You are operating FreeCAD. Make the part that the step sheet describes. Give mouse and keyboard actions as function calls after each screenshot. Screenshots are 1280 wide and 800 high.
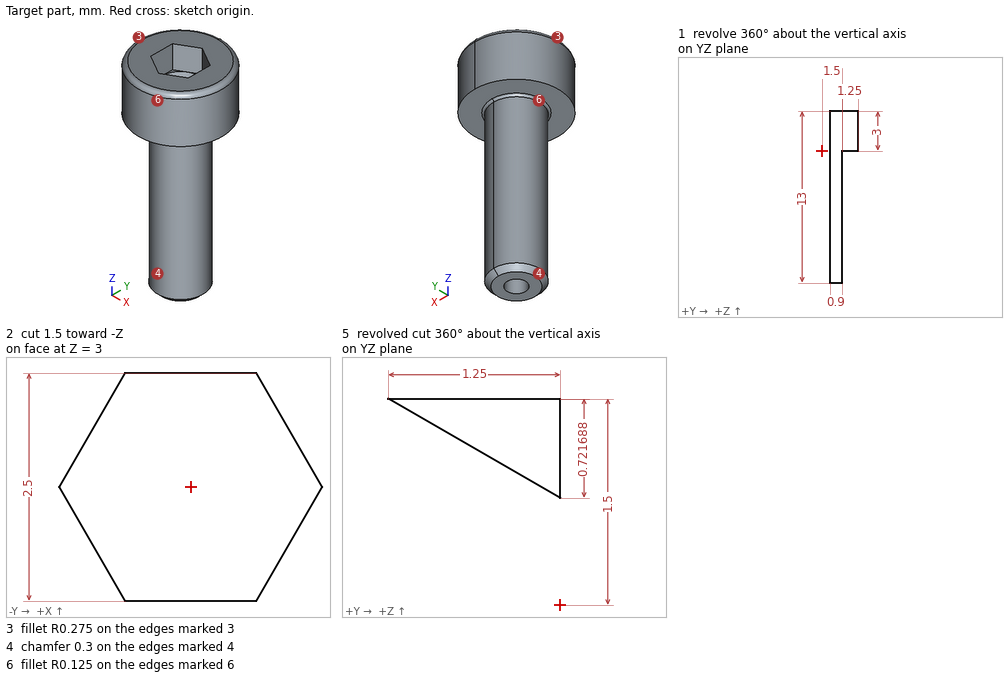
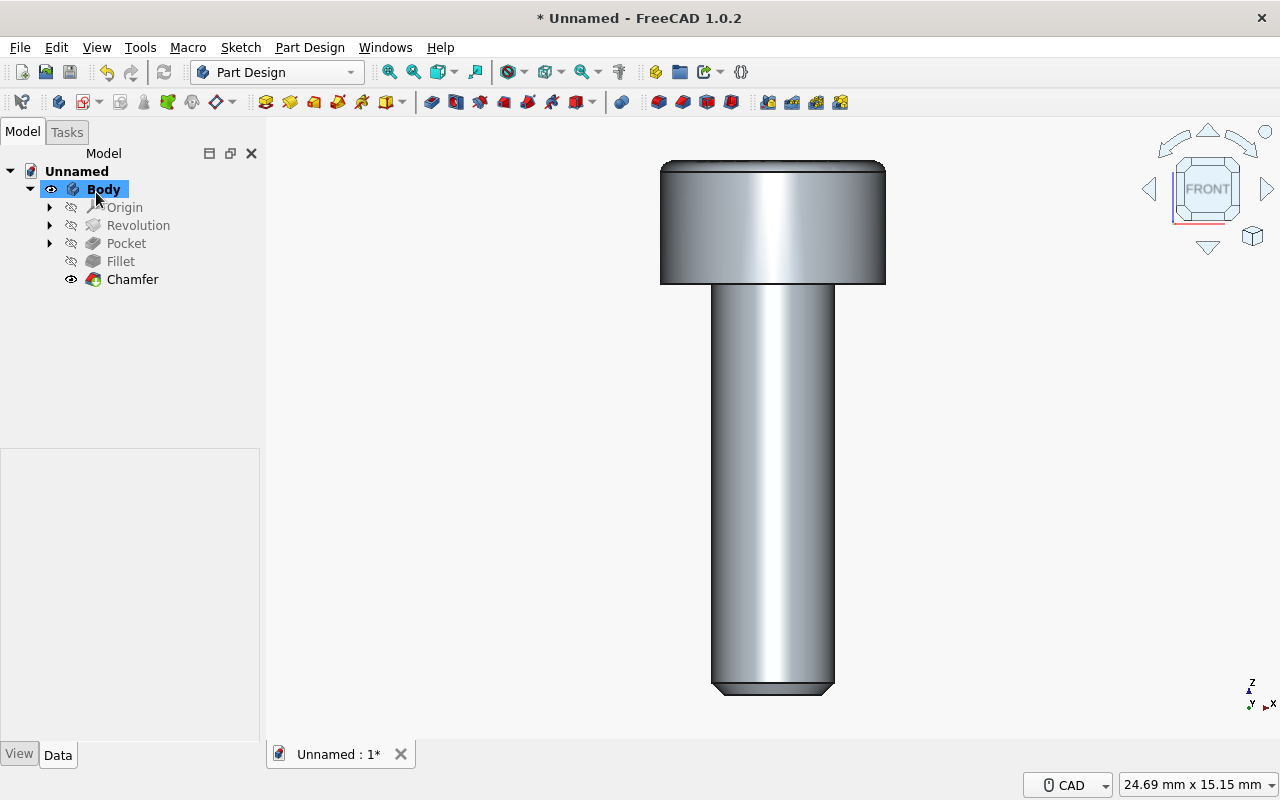
click(84, 102)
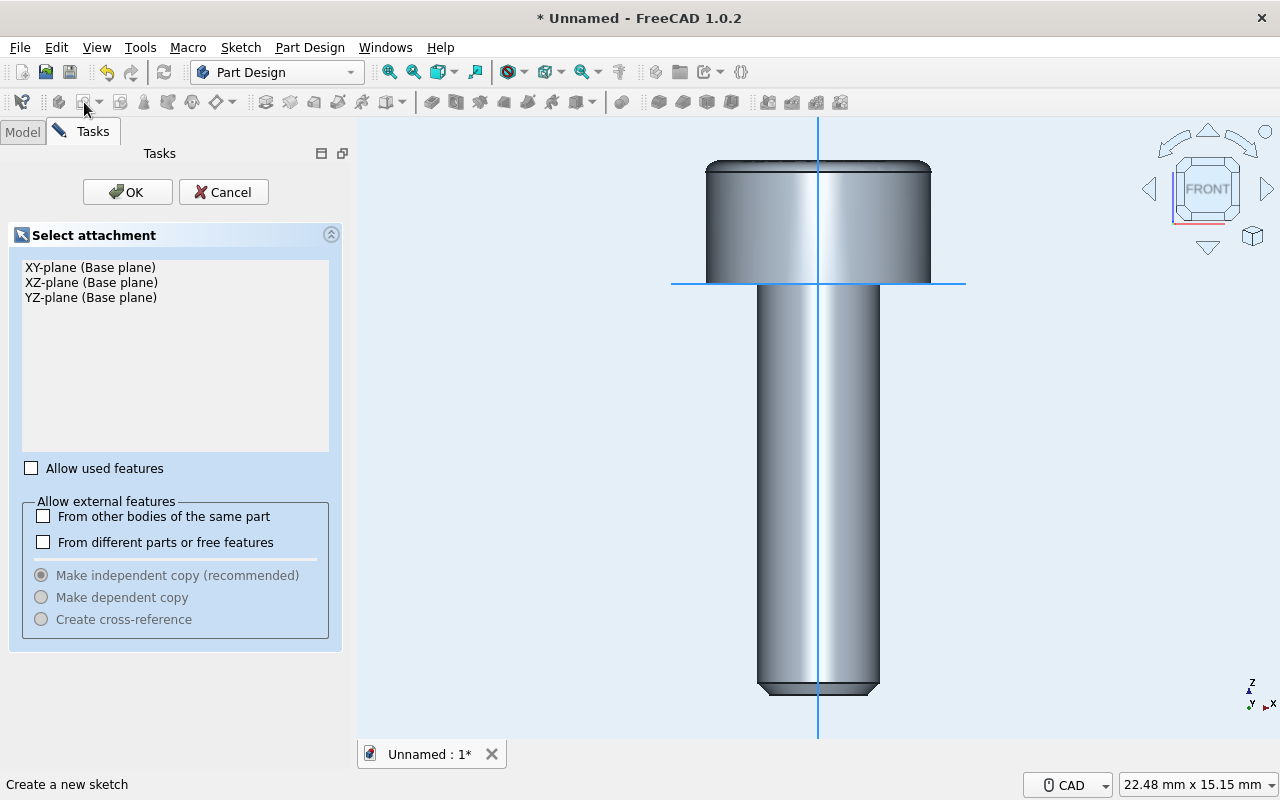
click(82, 298)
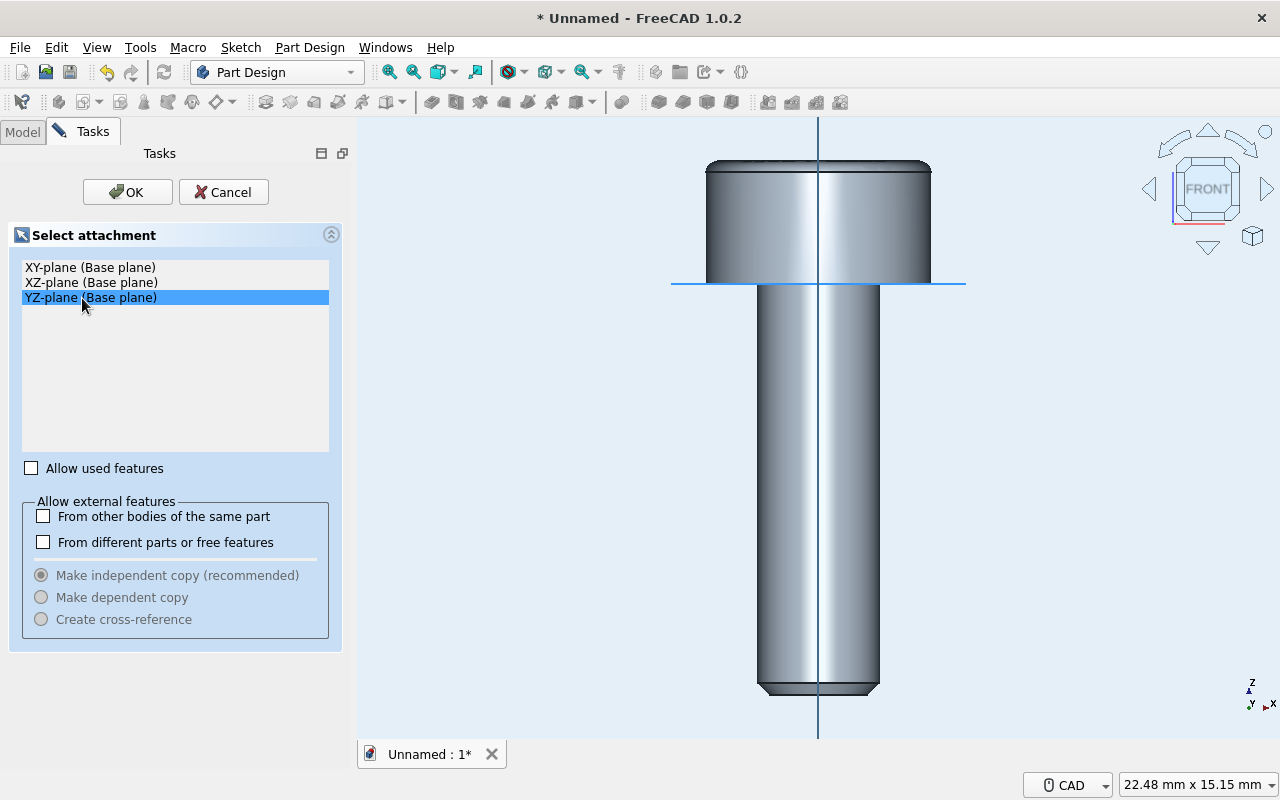
click(128, 192)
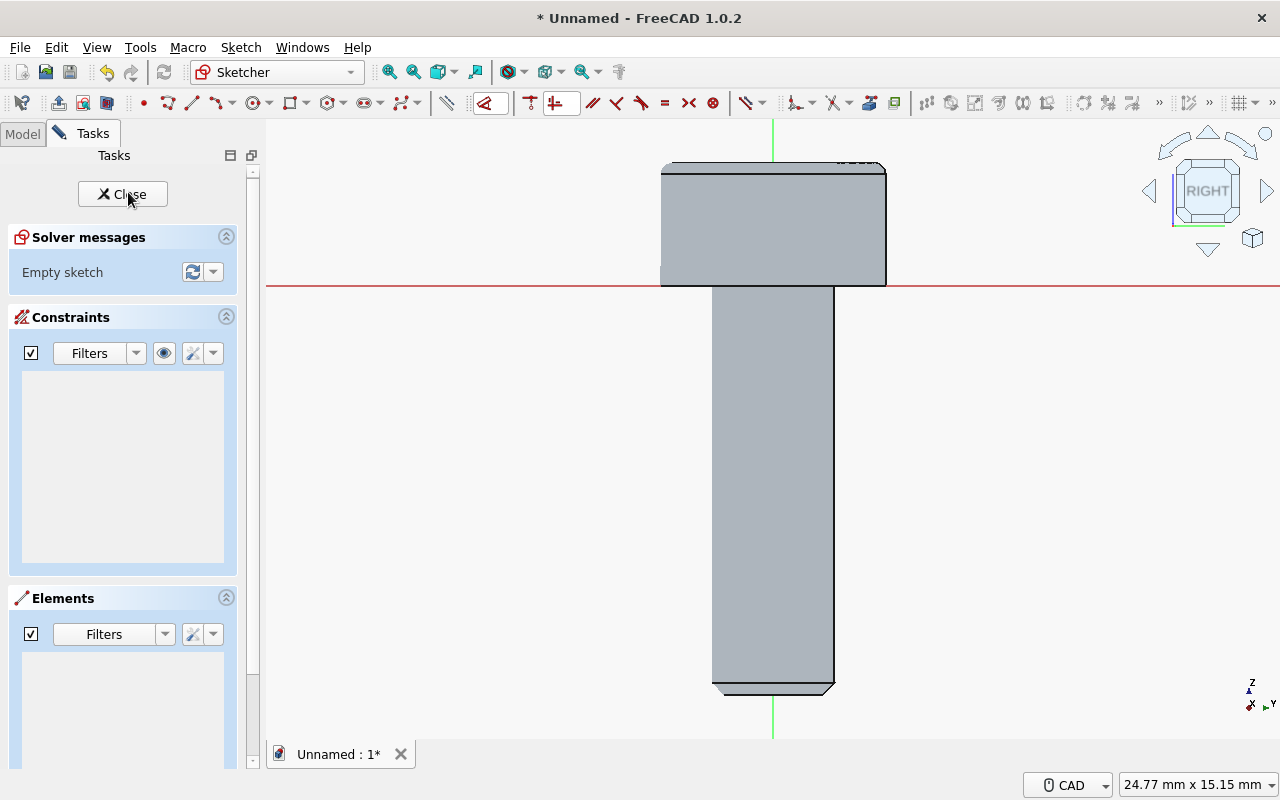
click(108, 104)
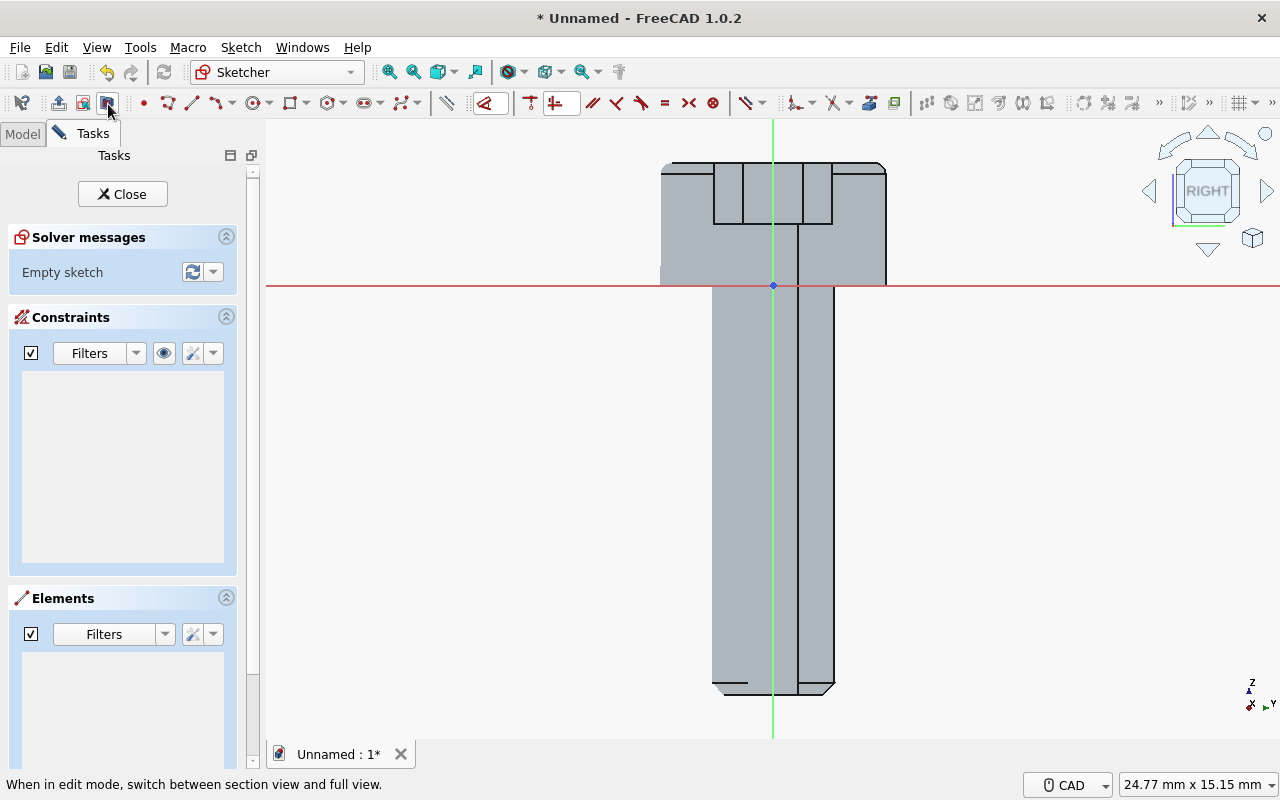
scroll(756, 221, up, 9)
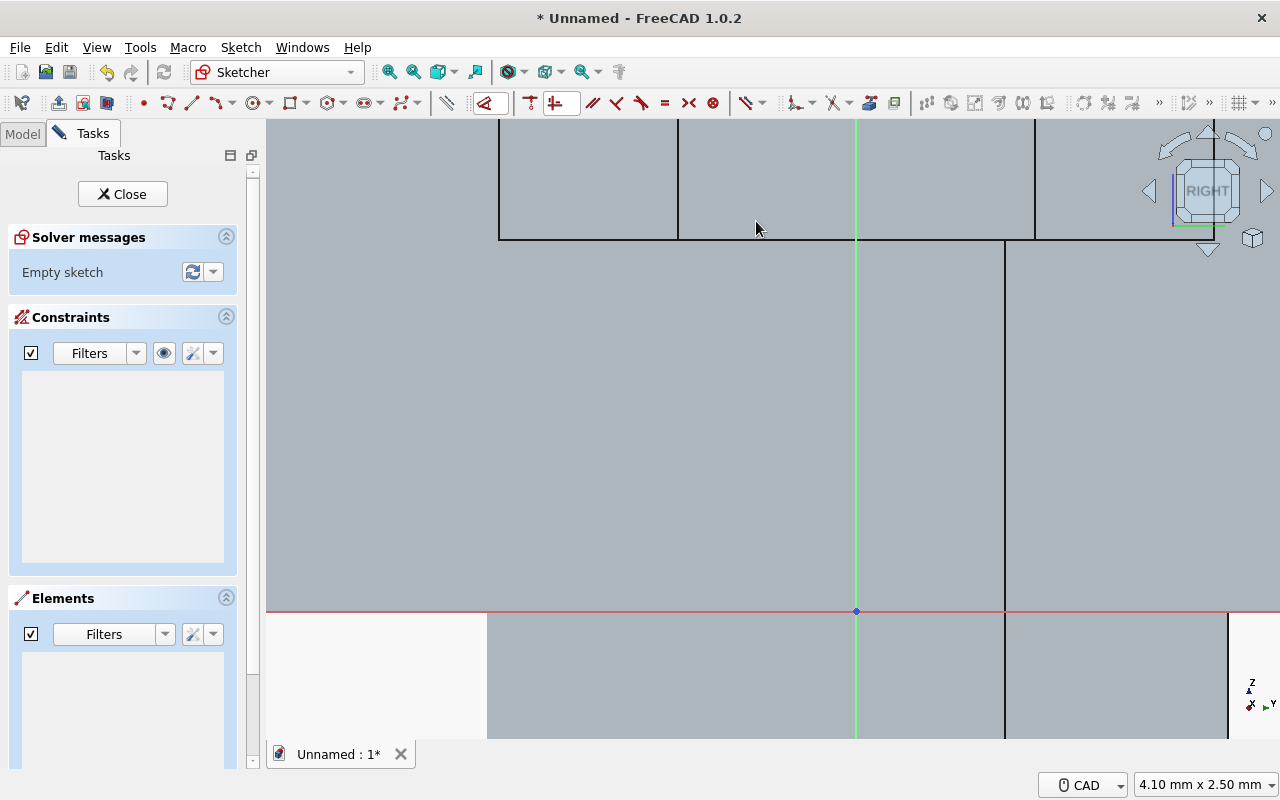
click(168, 104)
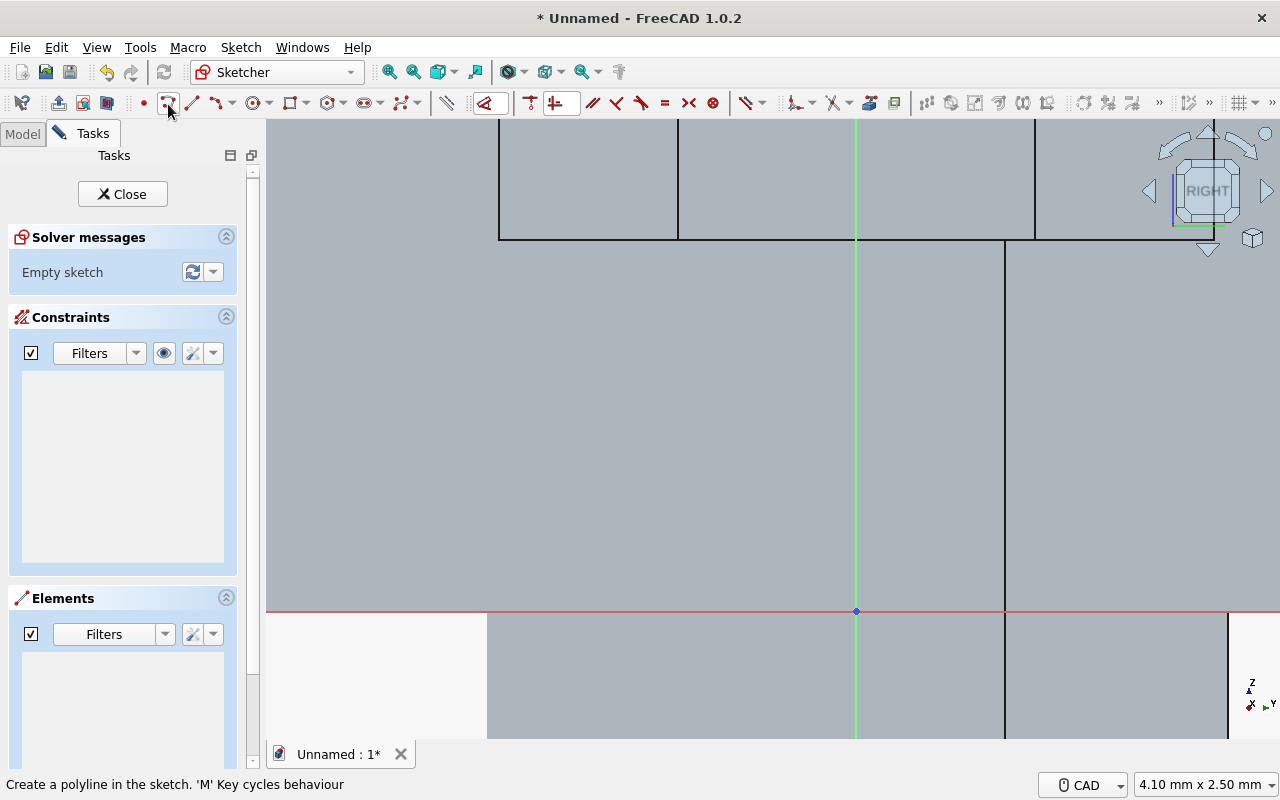
click(856, 419)
click(847, 240)
click(547, 240)
click(856, 420)
key(Escape)
key(Escape)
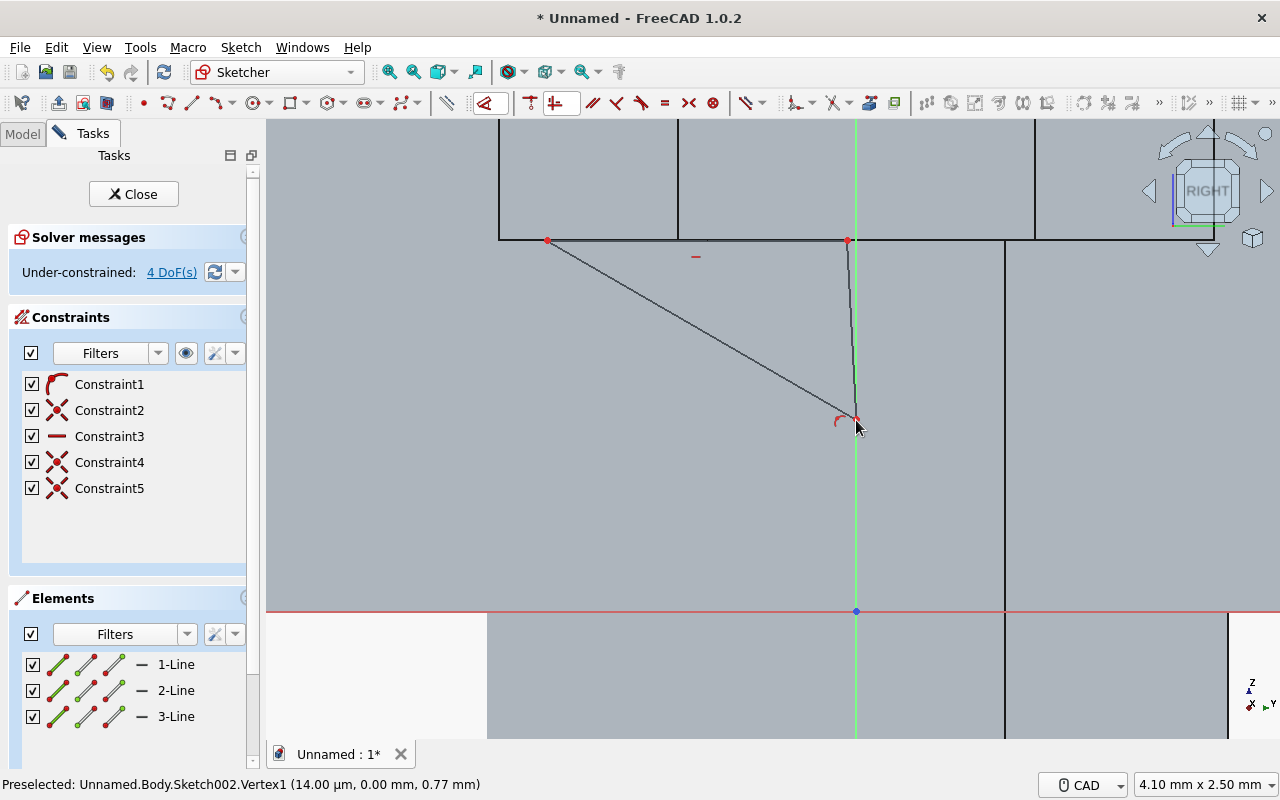
click(854, 366)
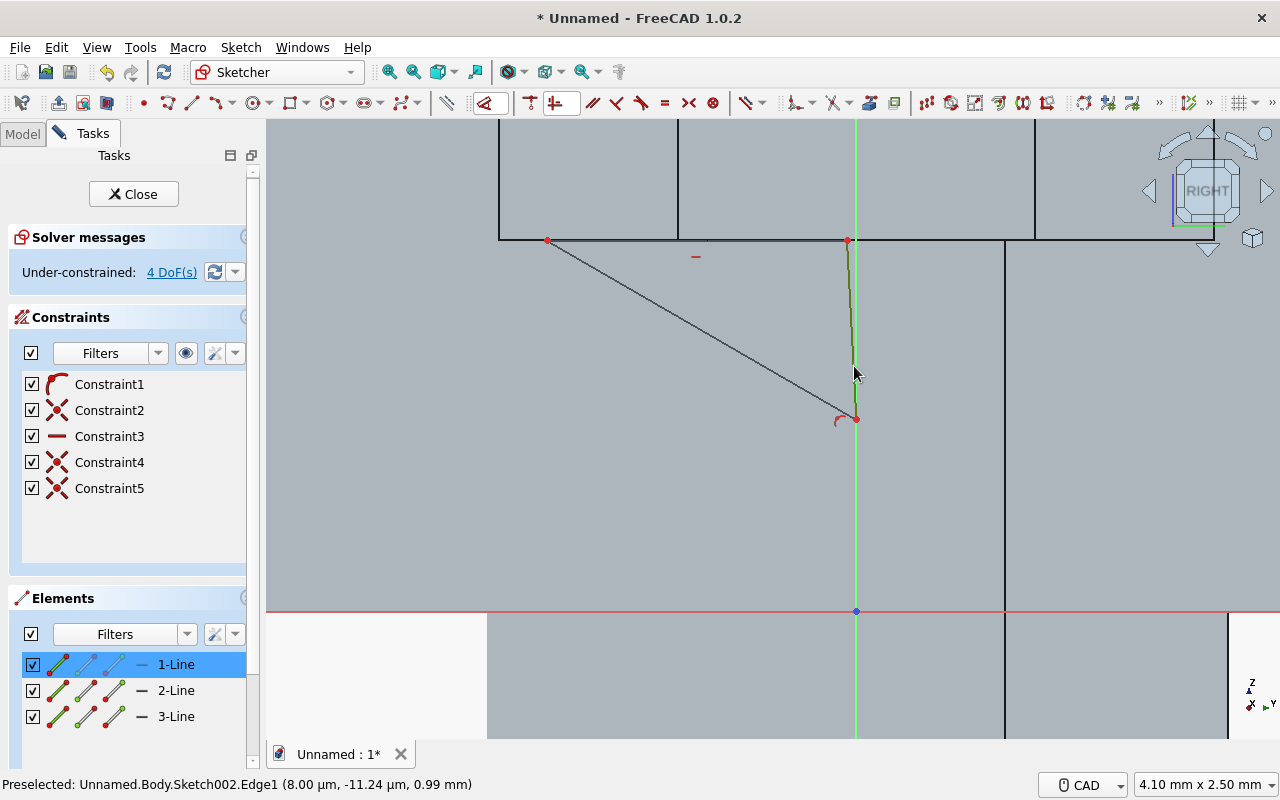
key(v)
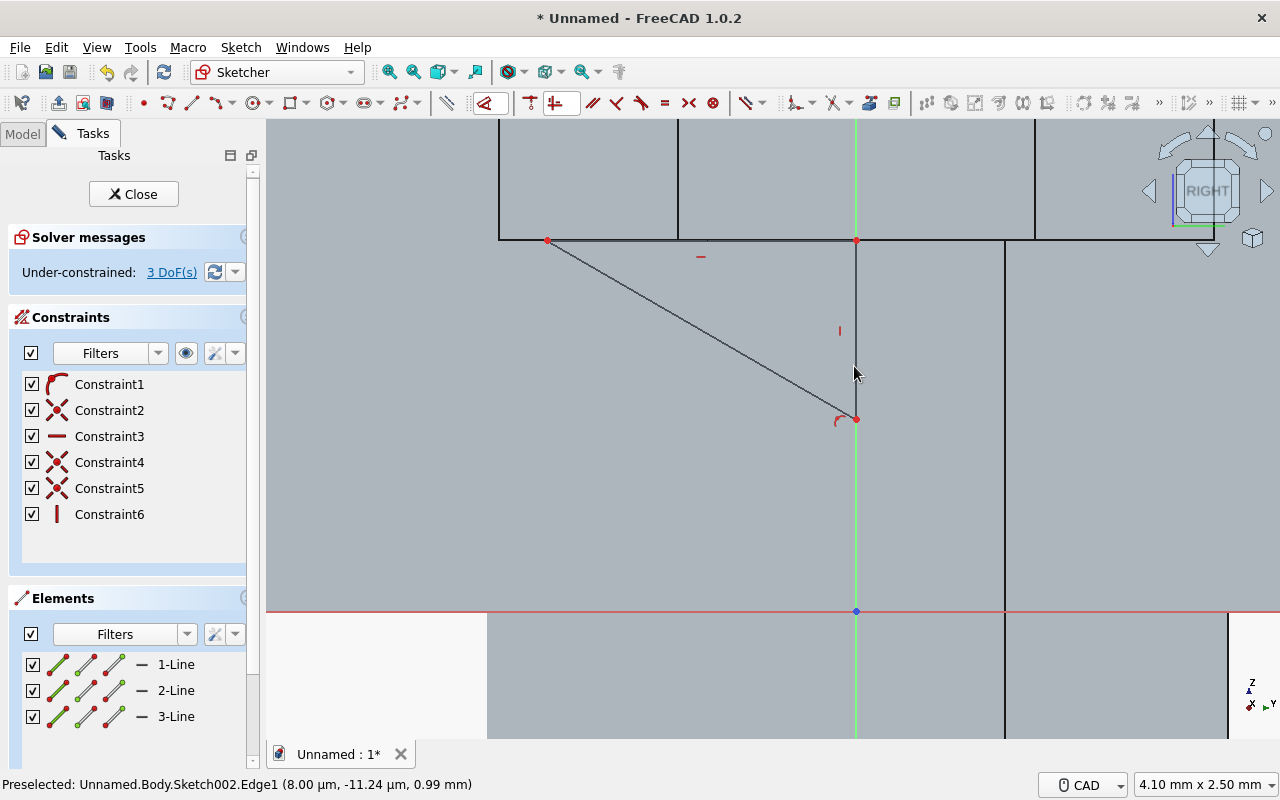
click(764, 241)